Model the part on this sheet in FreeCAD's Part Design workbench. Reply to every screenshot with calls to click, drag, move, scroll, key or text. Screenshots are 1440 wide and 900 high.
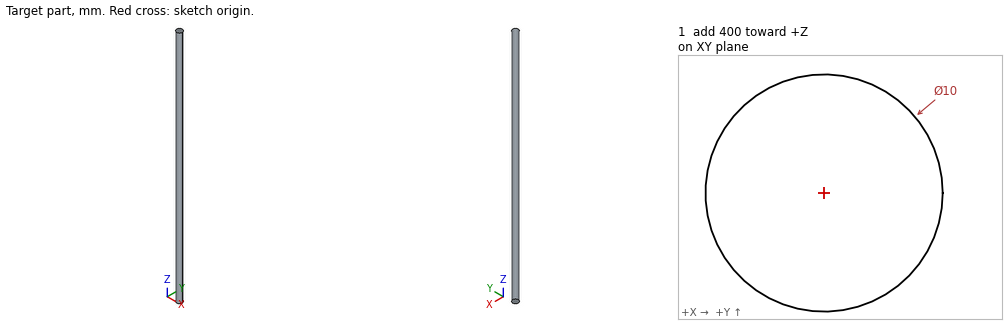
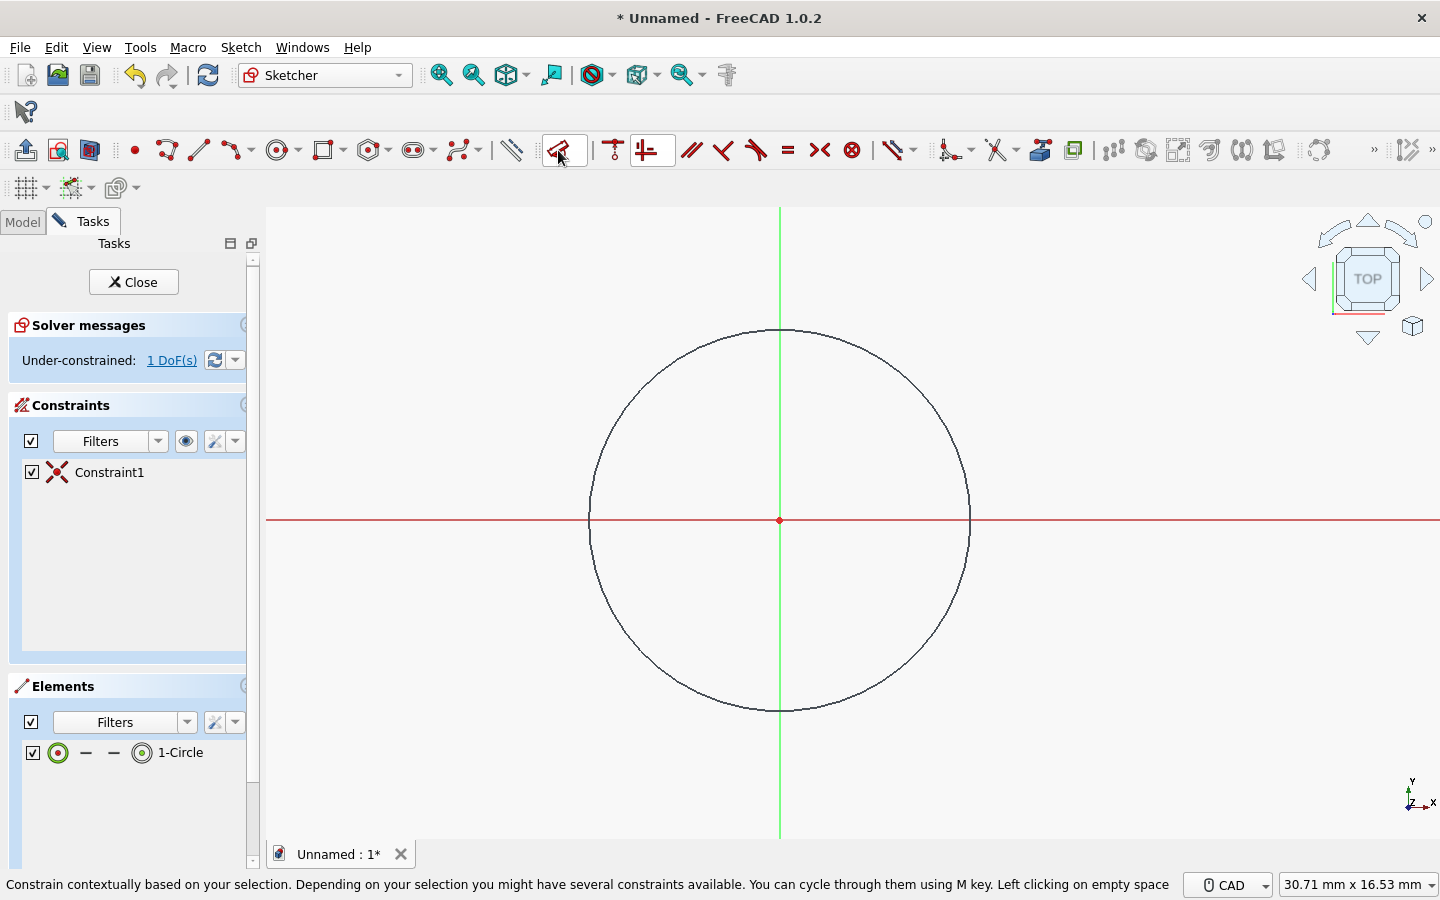
click(914, 385)
click(937, 362)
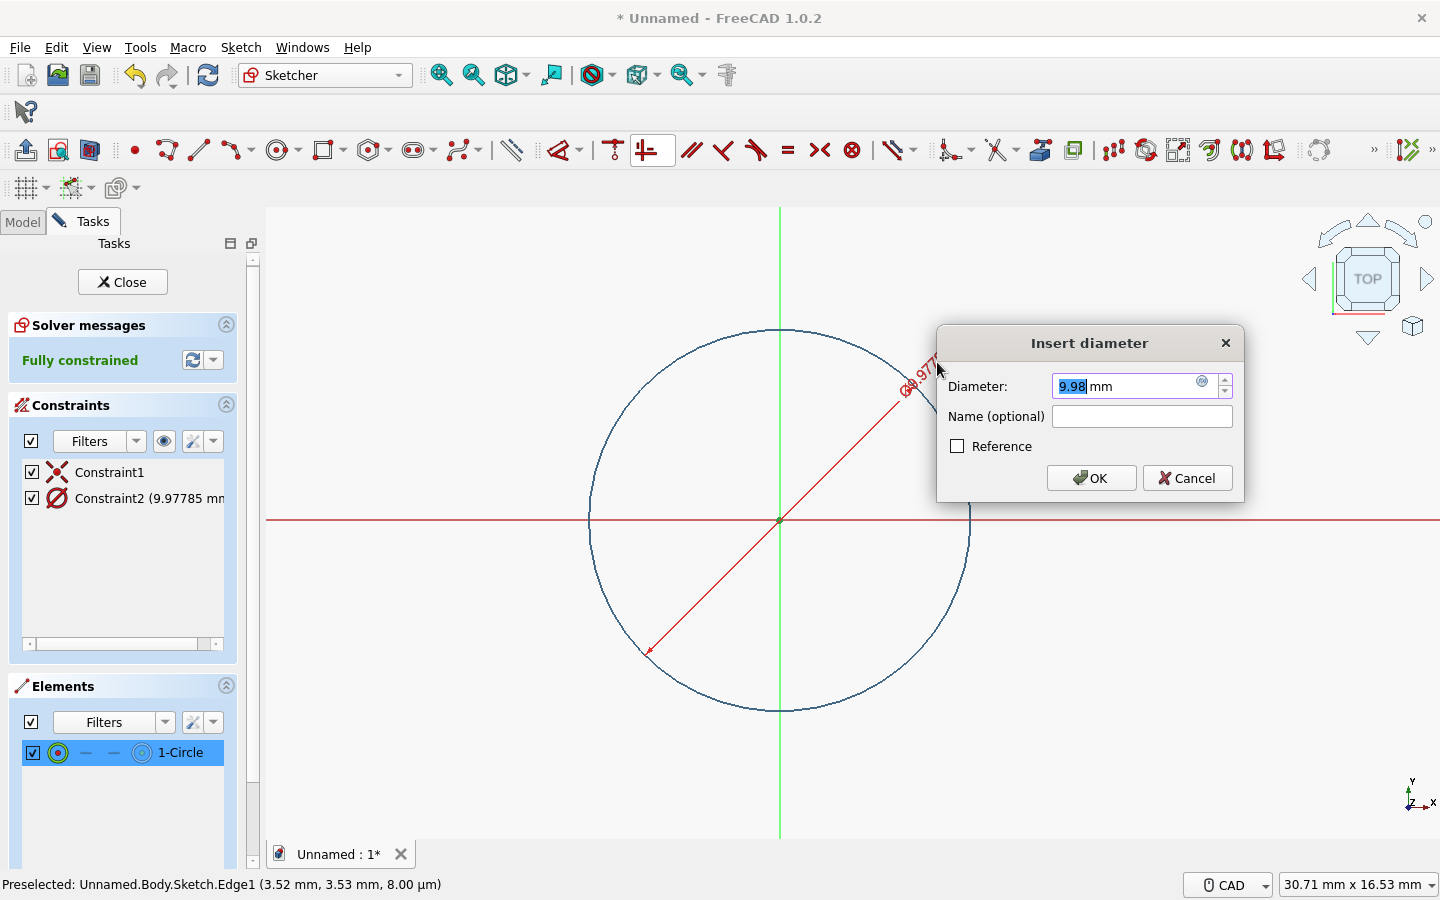
text(10)
key(Return)
key(Escape)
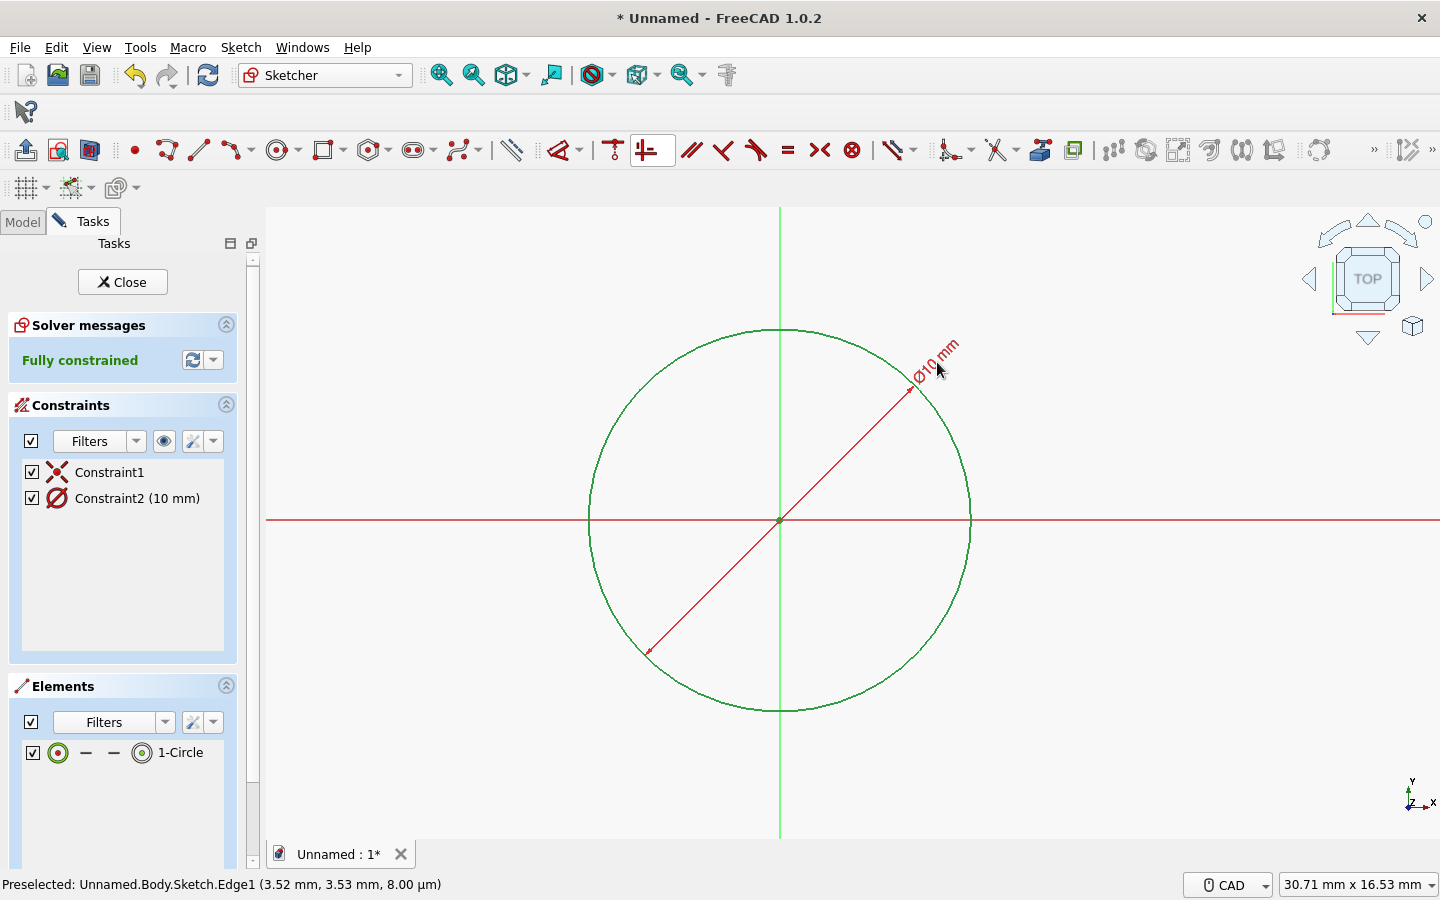
click(123, 282)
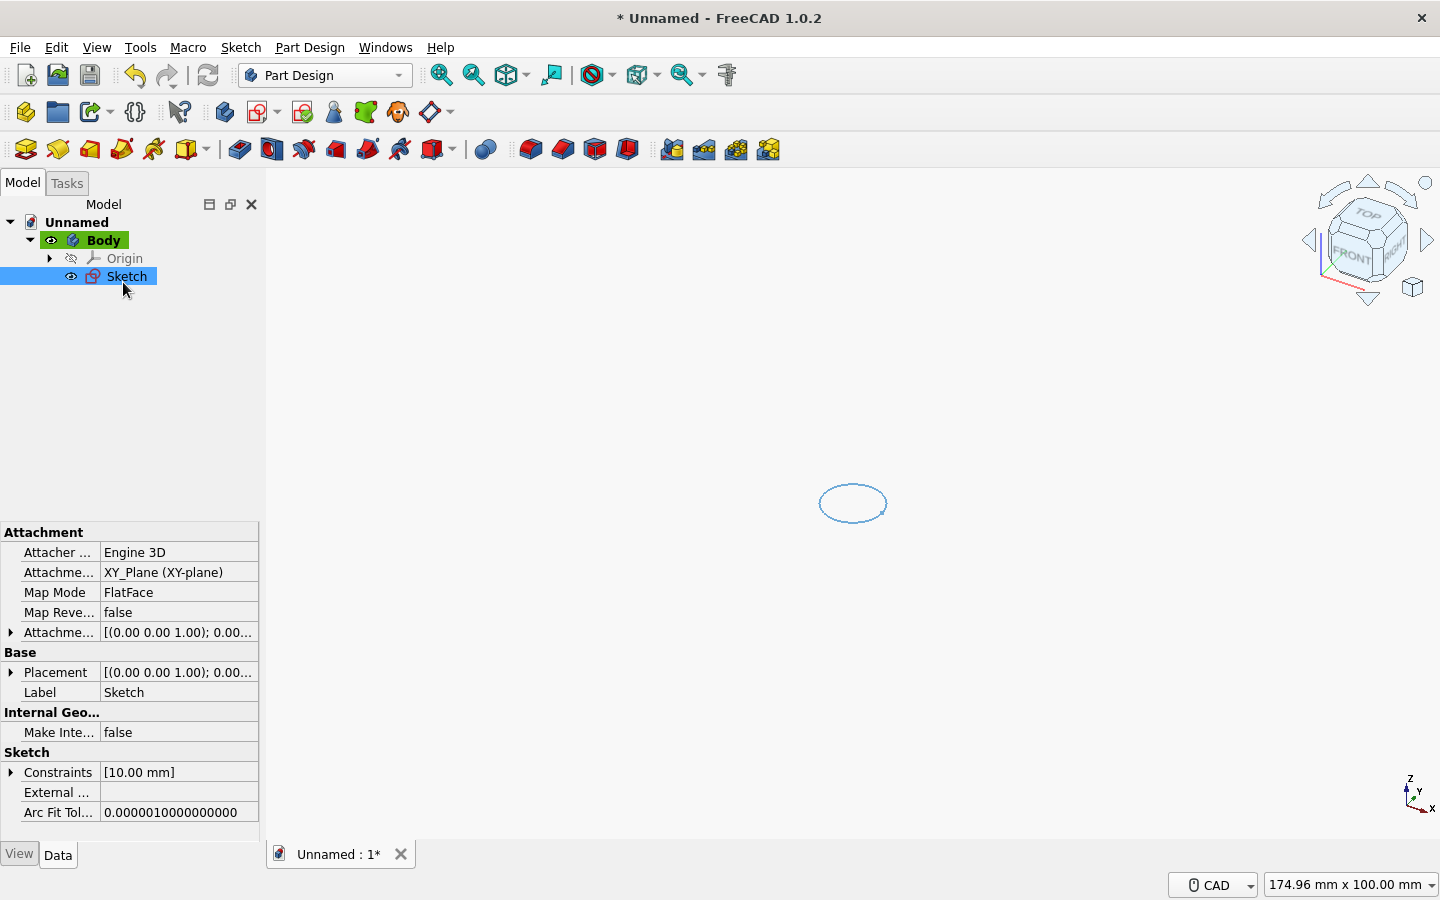
click(26, 150)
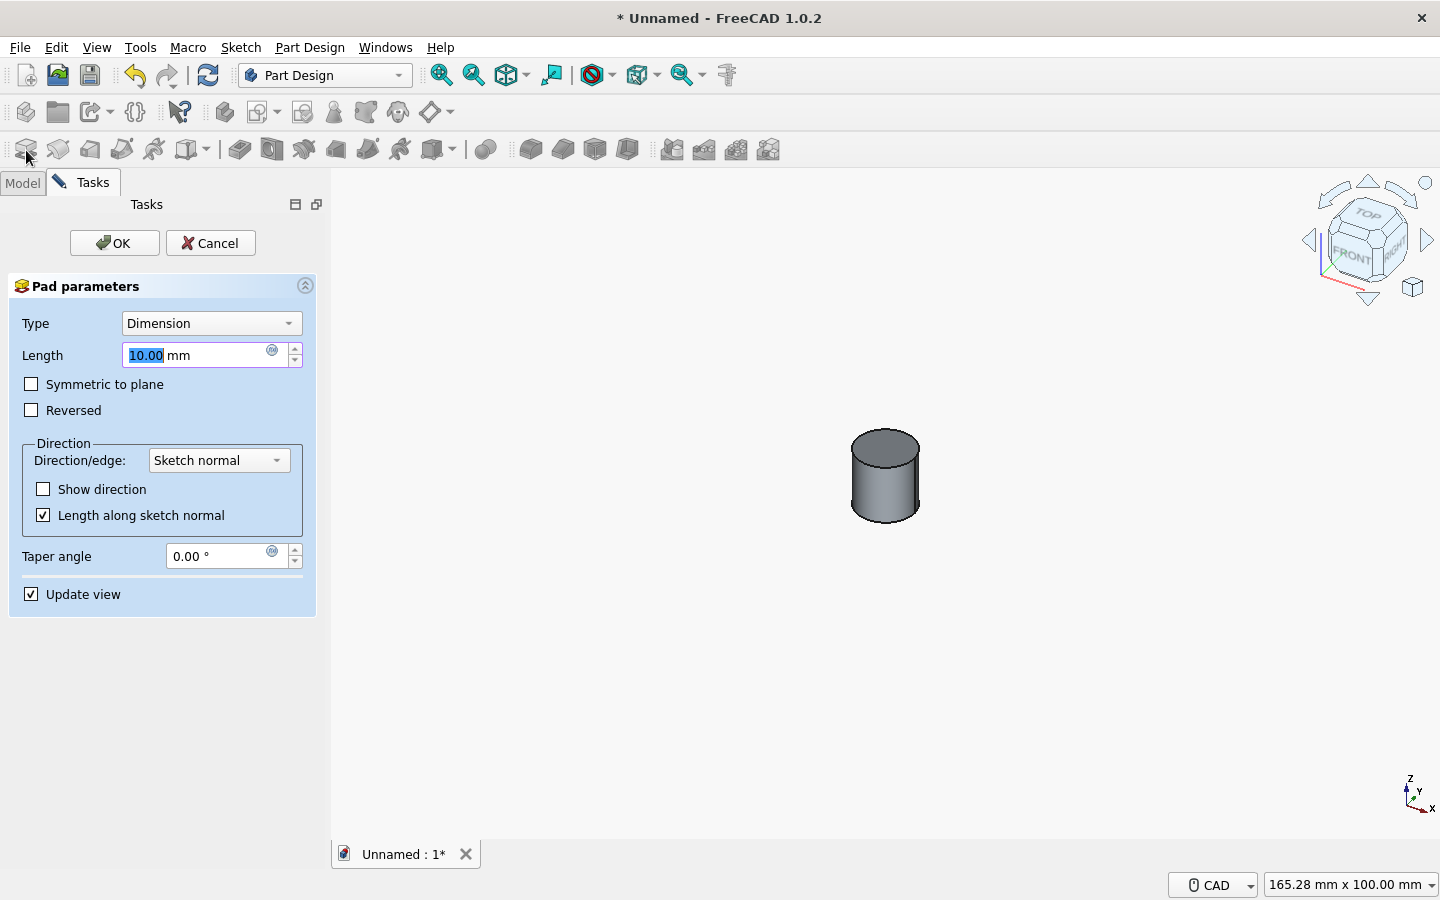
text(400)
key(Tab)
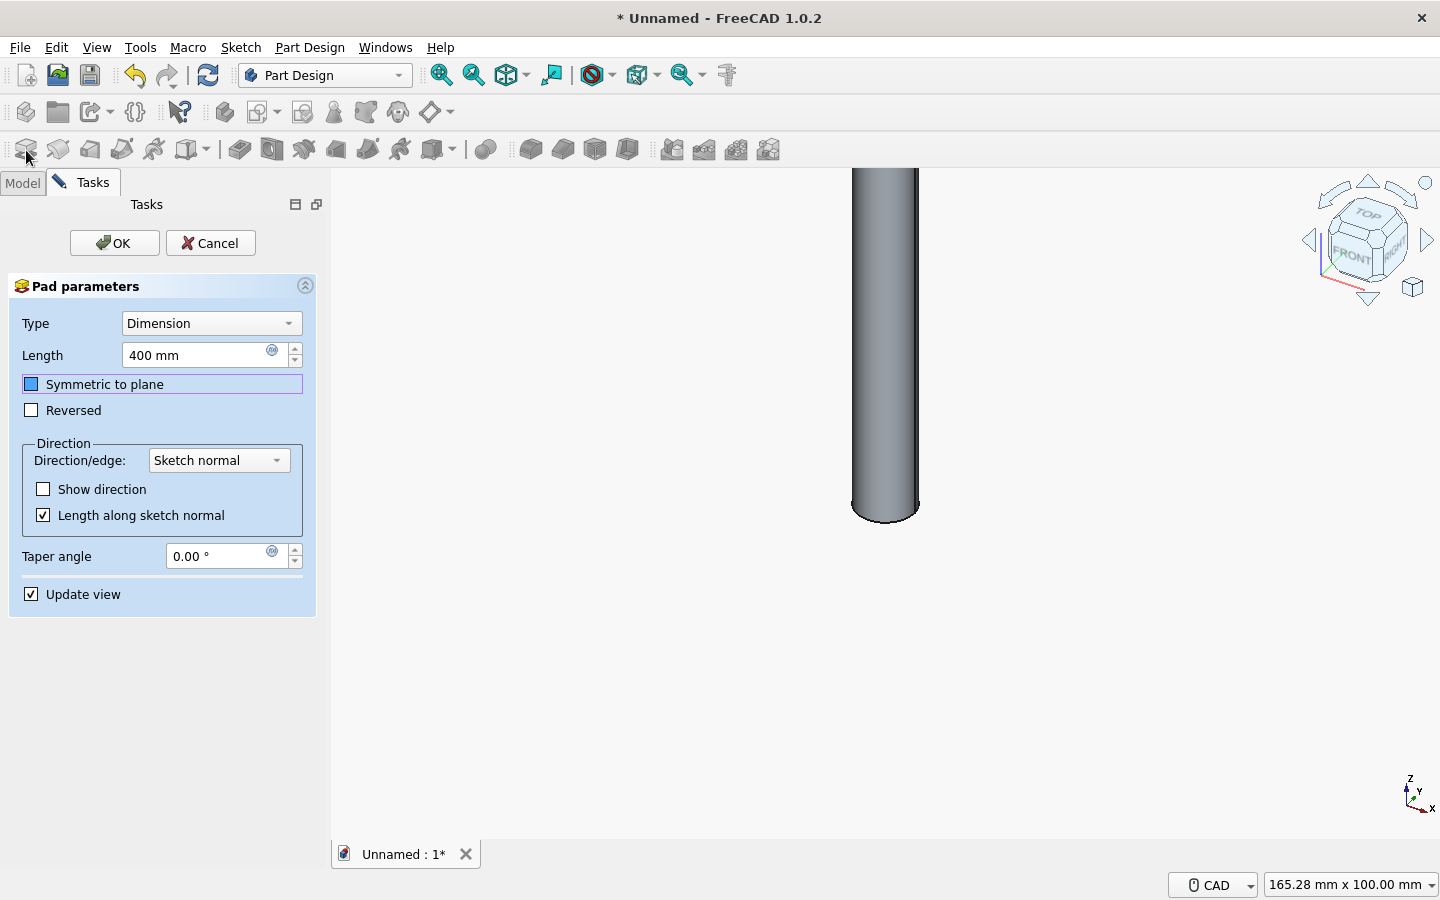
click(115, 243)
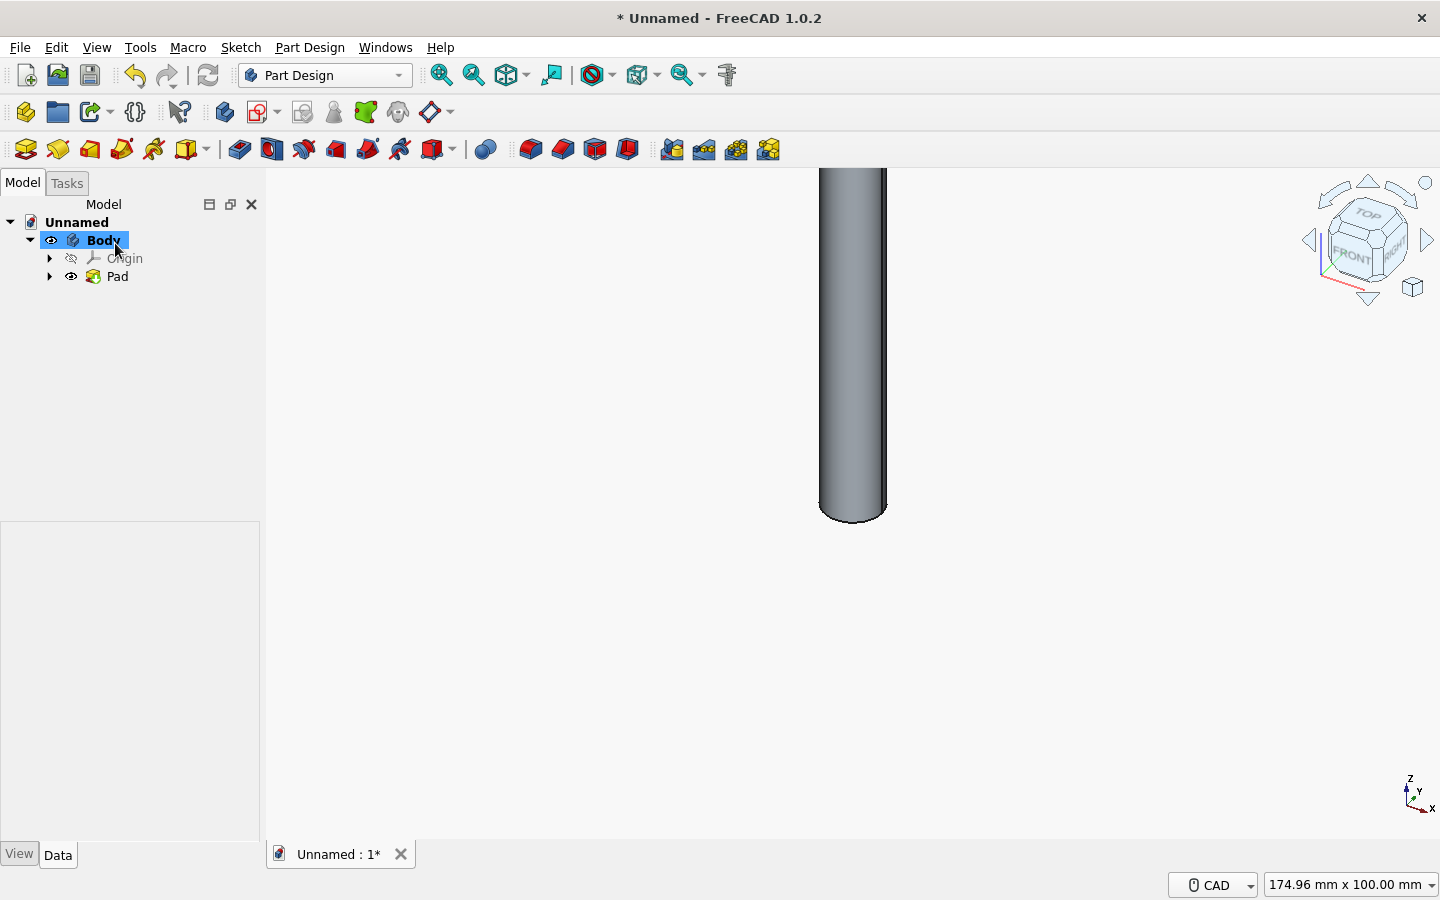
key(0)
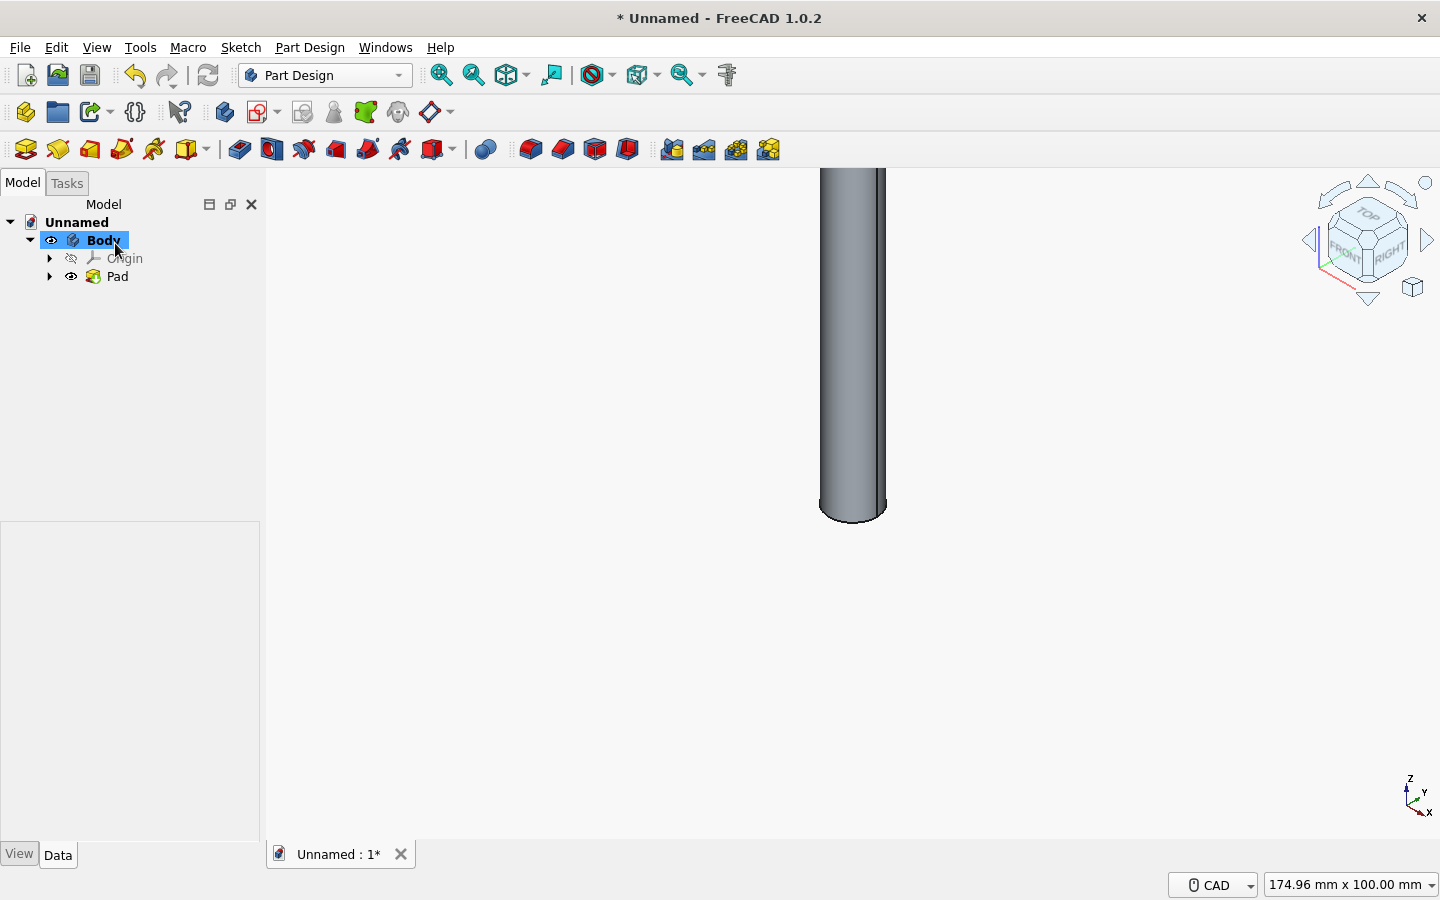
click(442, 76)